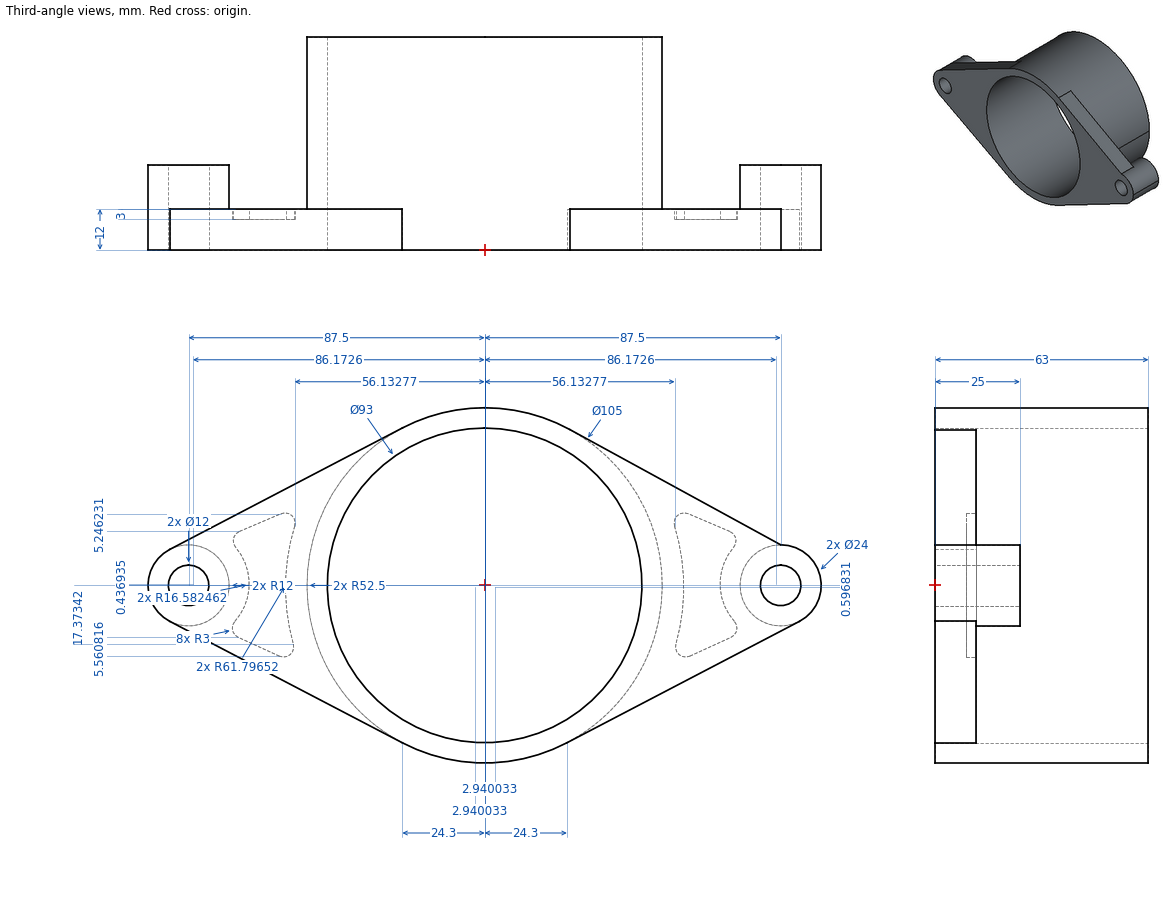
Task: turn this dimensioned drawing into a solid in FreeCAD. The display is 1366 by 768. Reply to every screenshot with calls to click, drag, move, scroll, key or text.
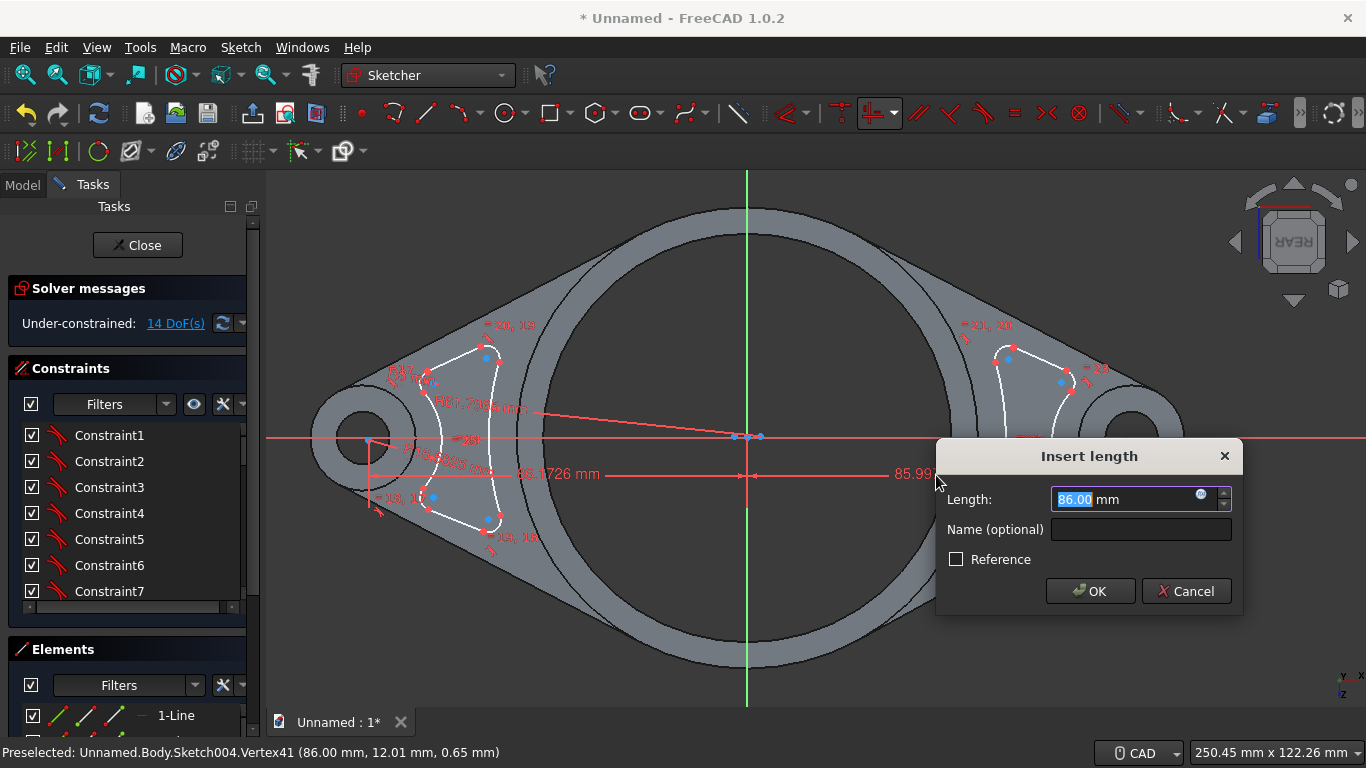
text(86.1726)
key(Return)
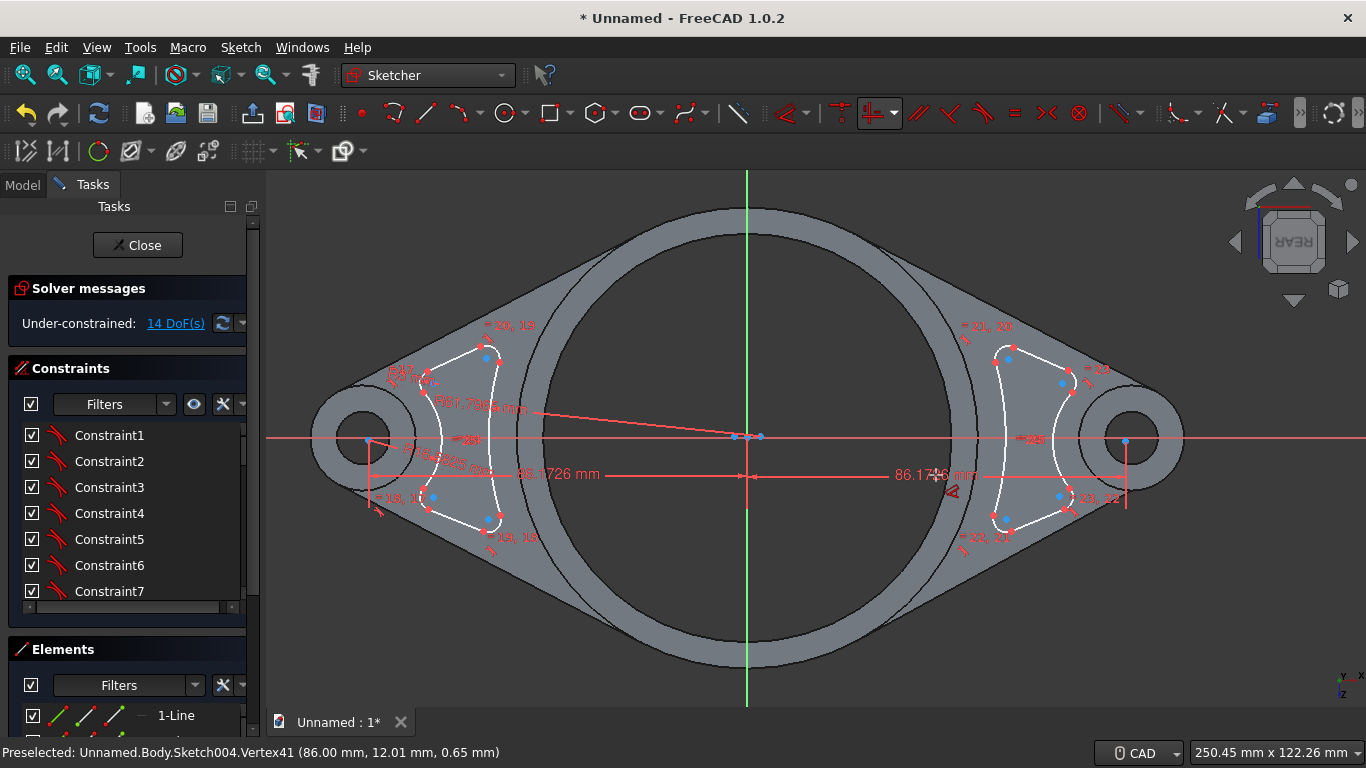
click(501, 515)
click(624, 549)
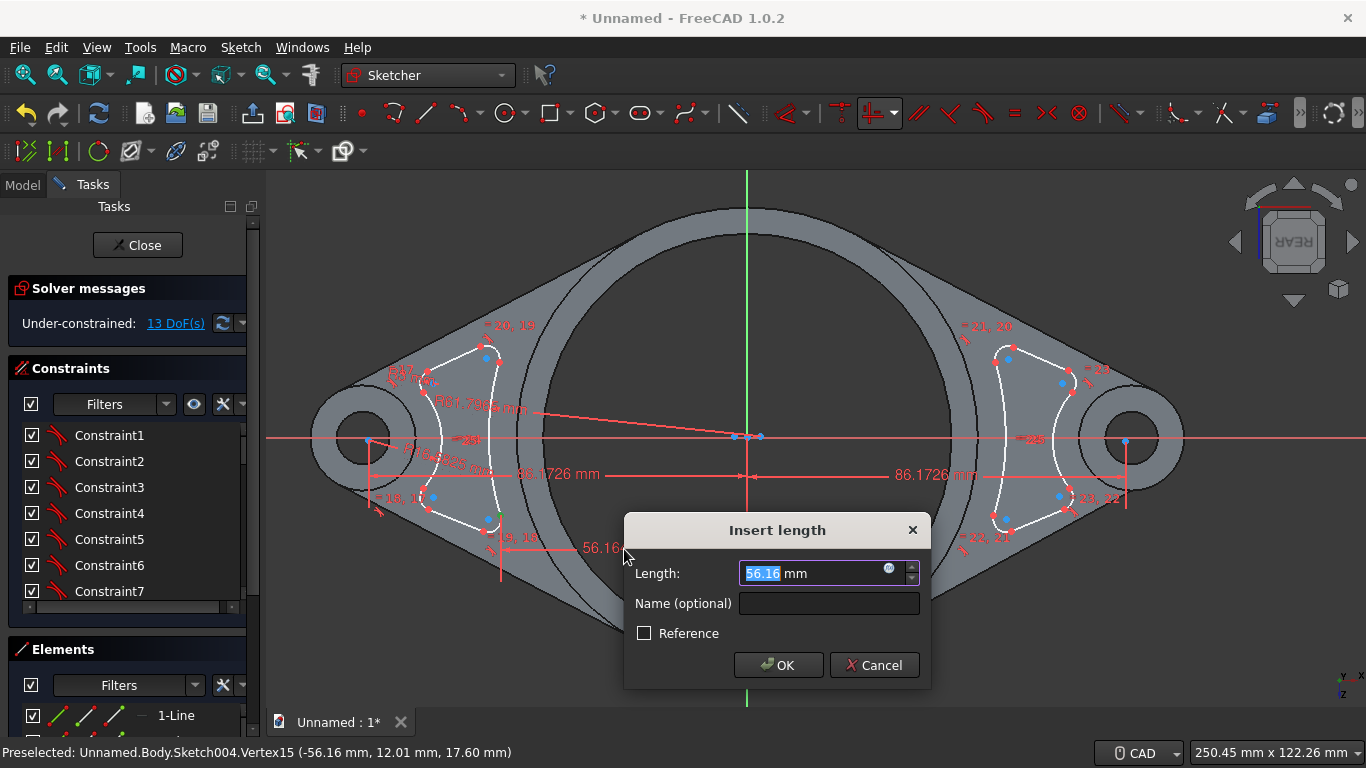
text(56.13277)
key(Return)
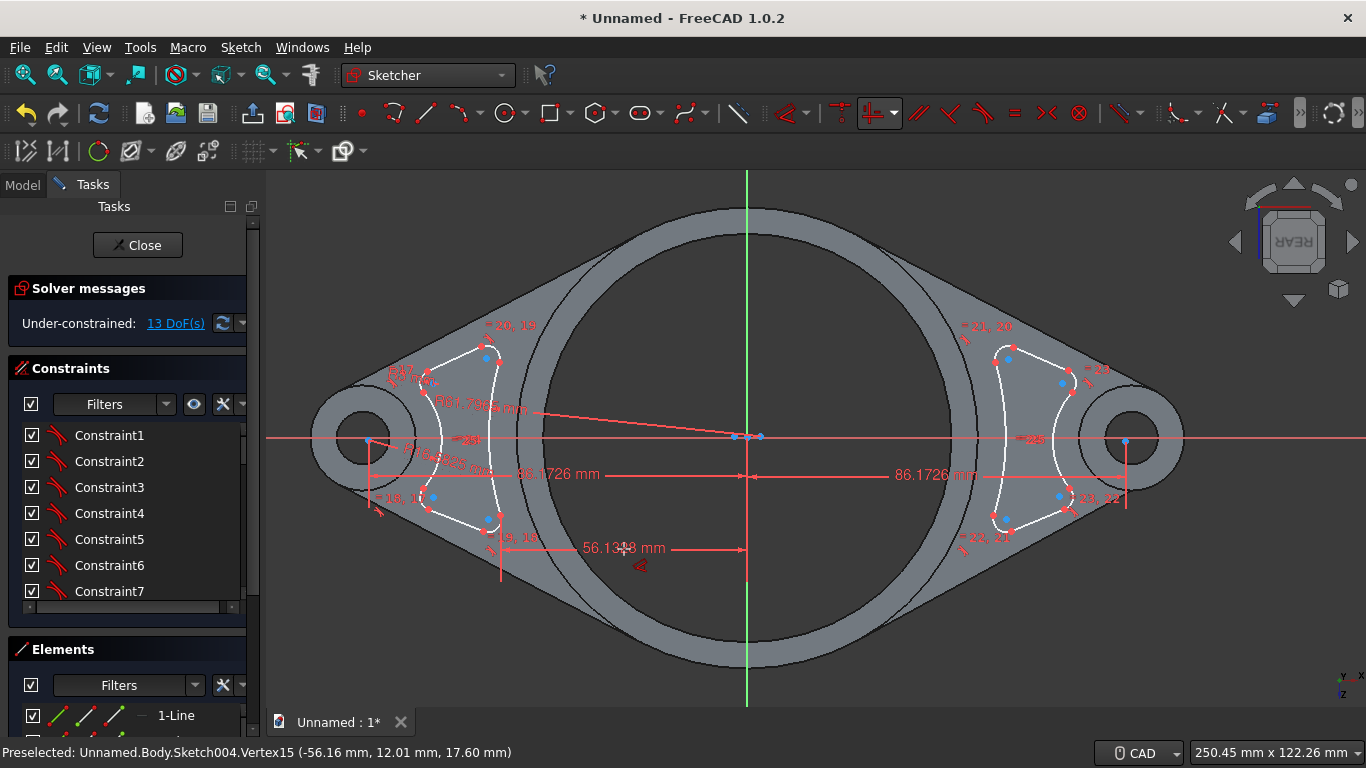
click(499, 362)
click(781, 400)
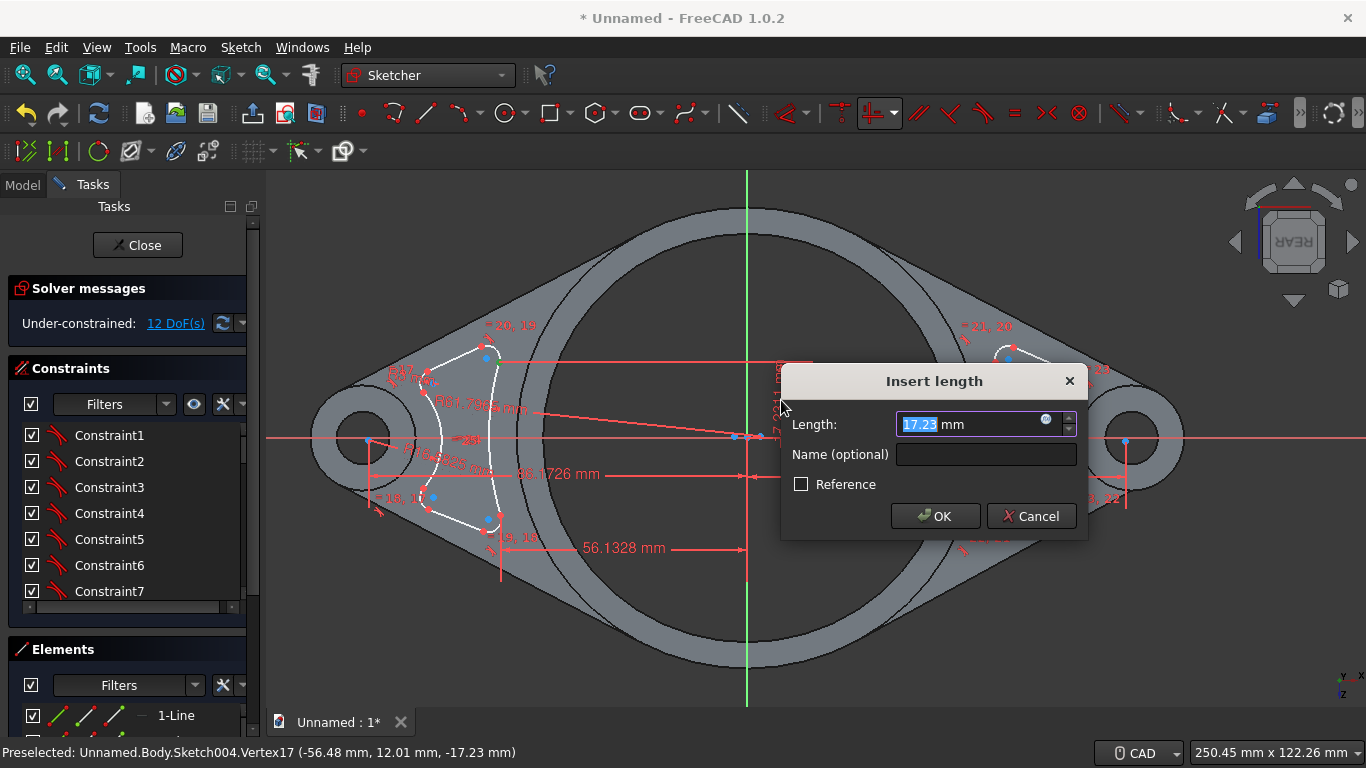
text(17.37342)
key(Return)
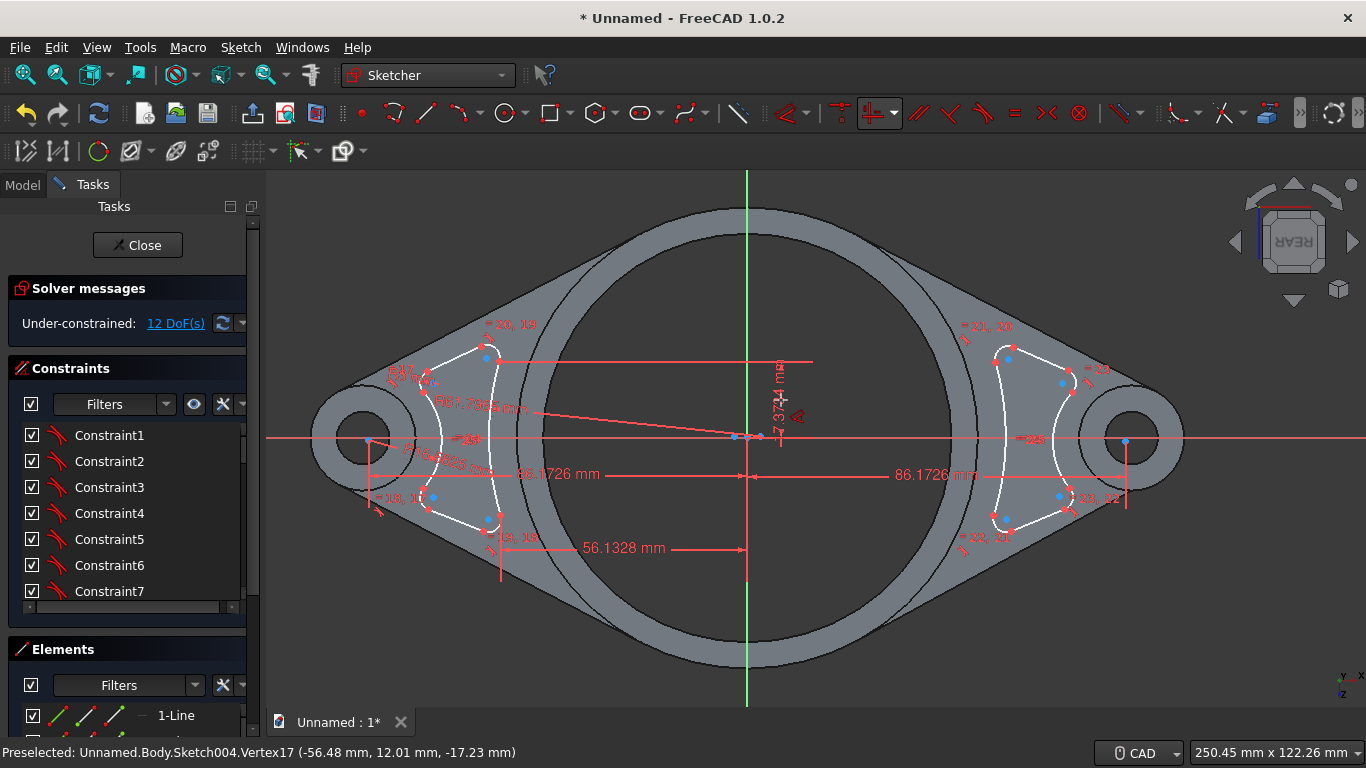
click(996, 363)
click(1030, 400)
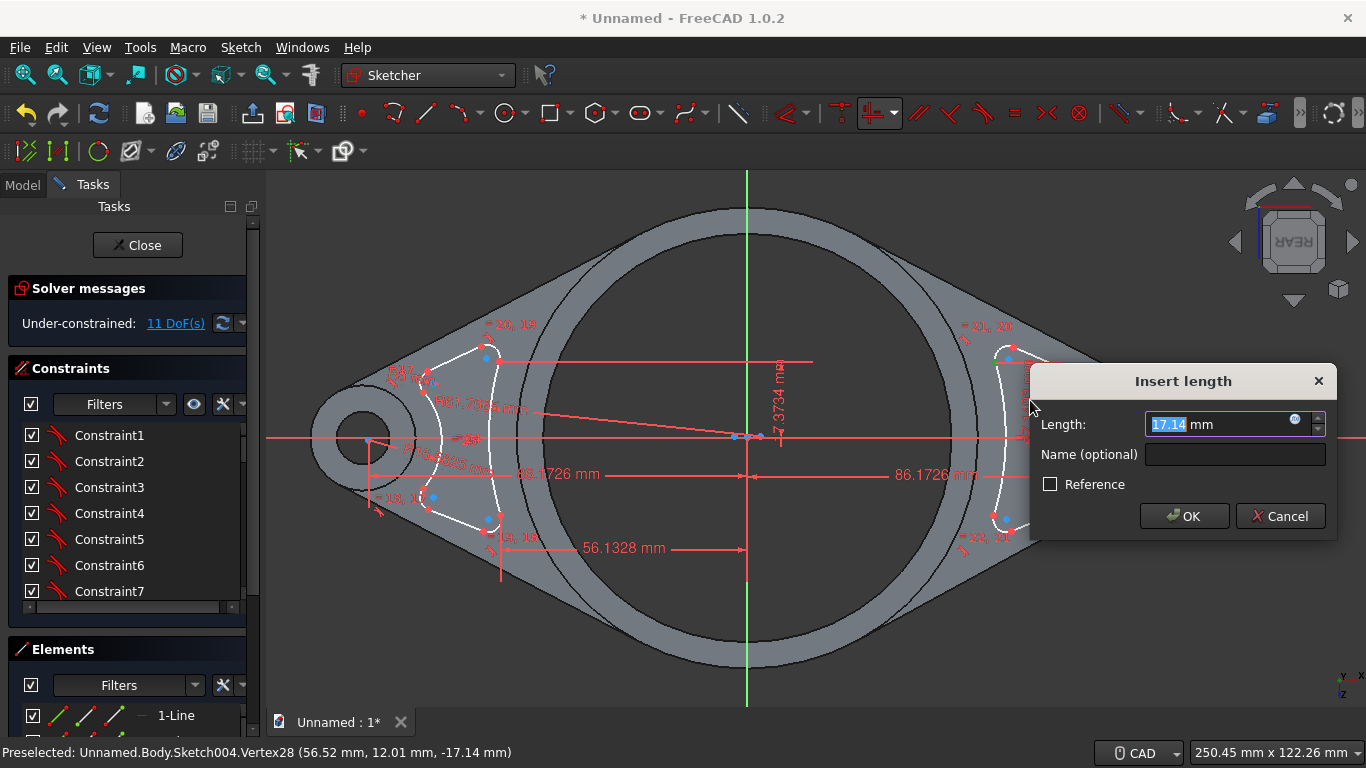
text(17.37342)
key(Return)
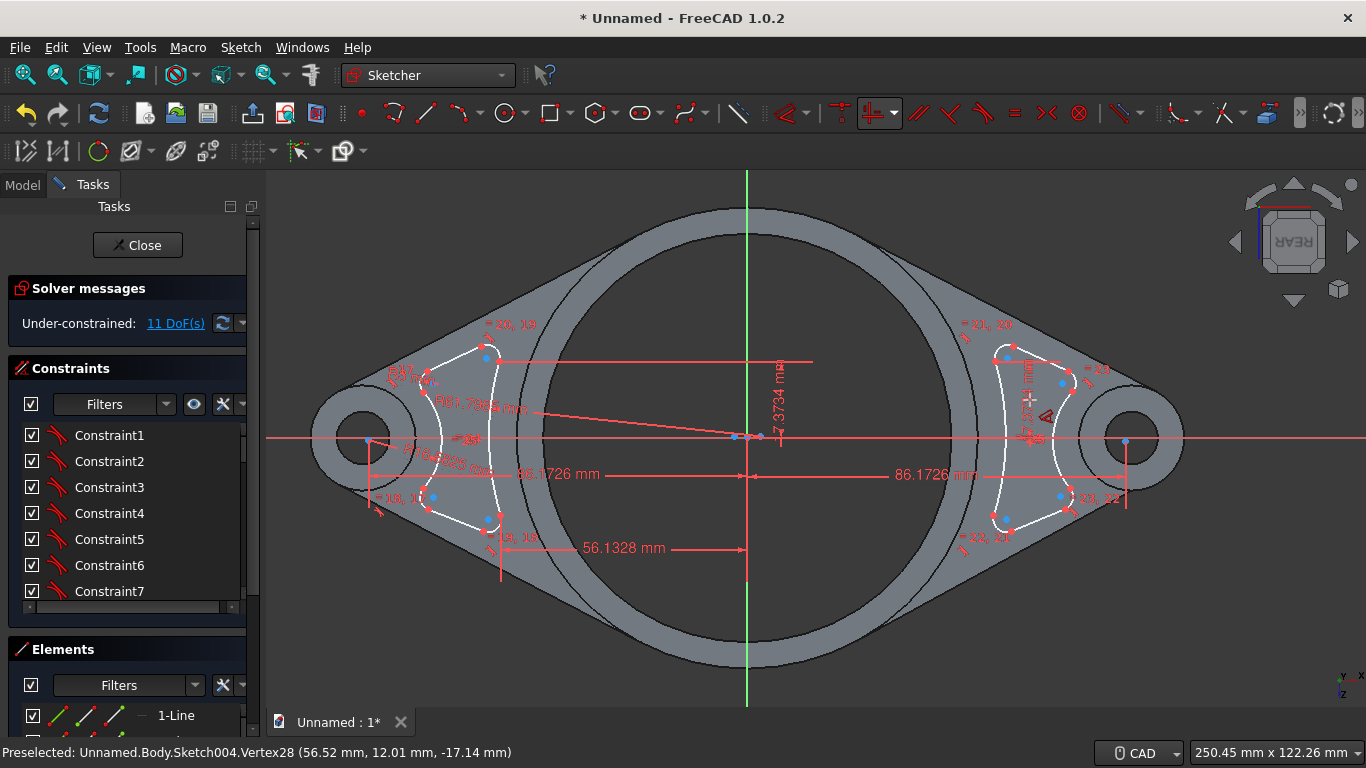
click(994, 515)
click(871, 549)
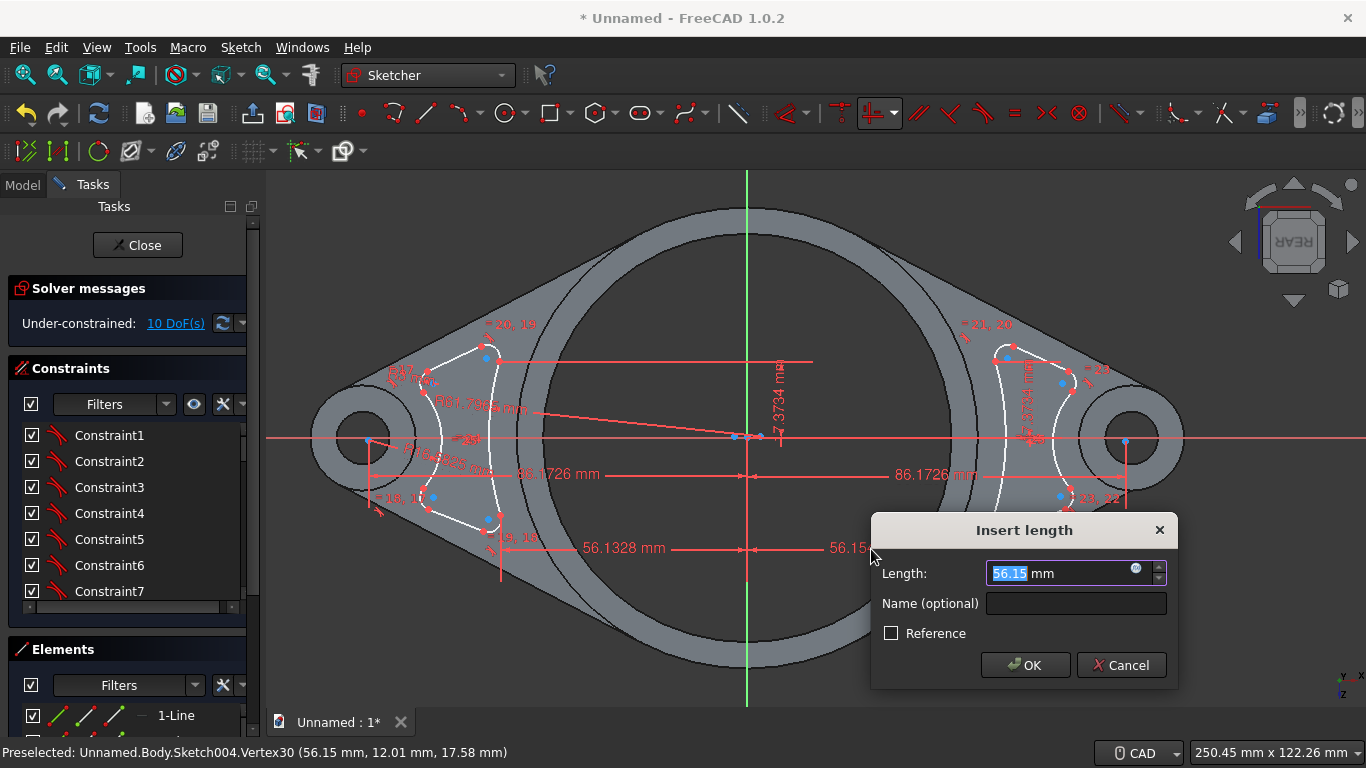
text(56.13277)
key(Return)